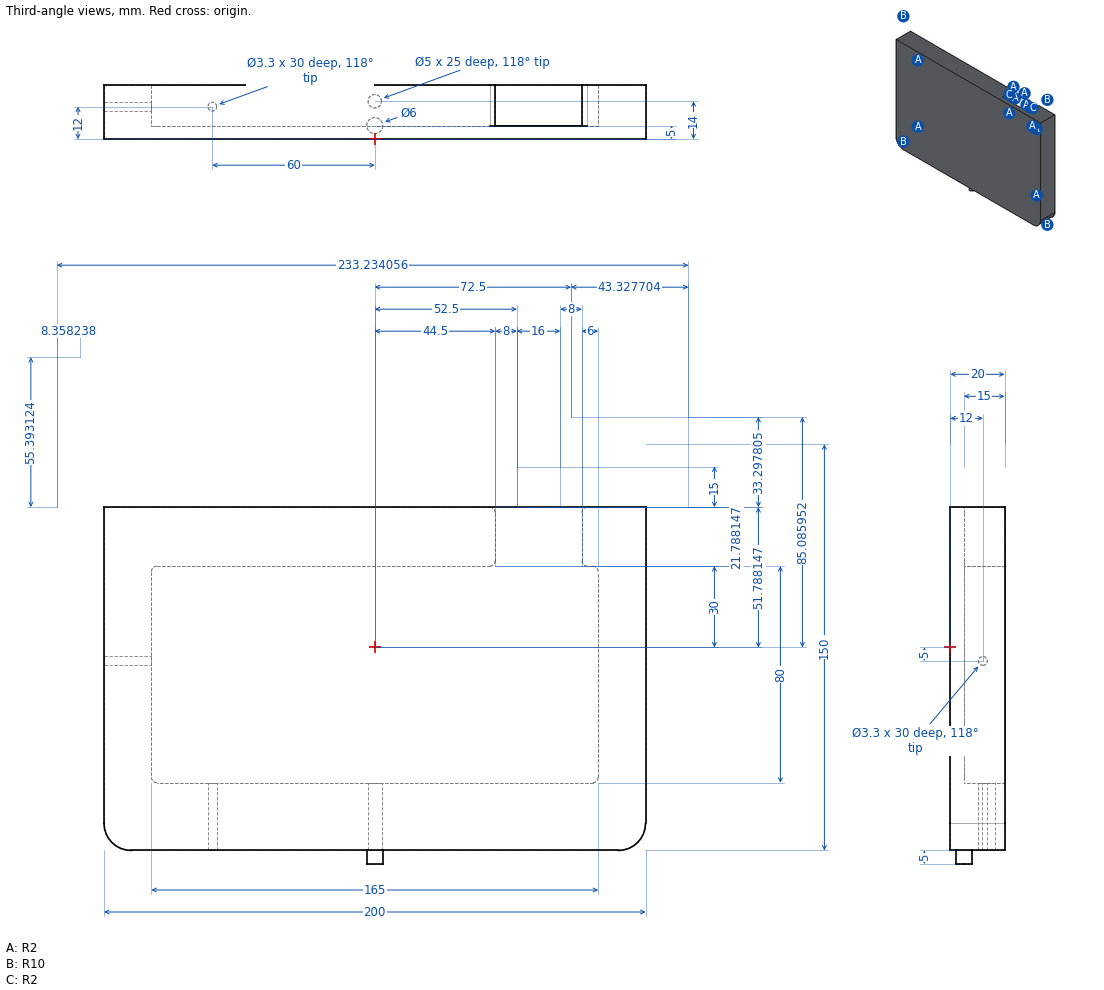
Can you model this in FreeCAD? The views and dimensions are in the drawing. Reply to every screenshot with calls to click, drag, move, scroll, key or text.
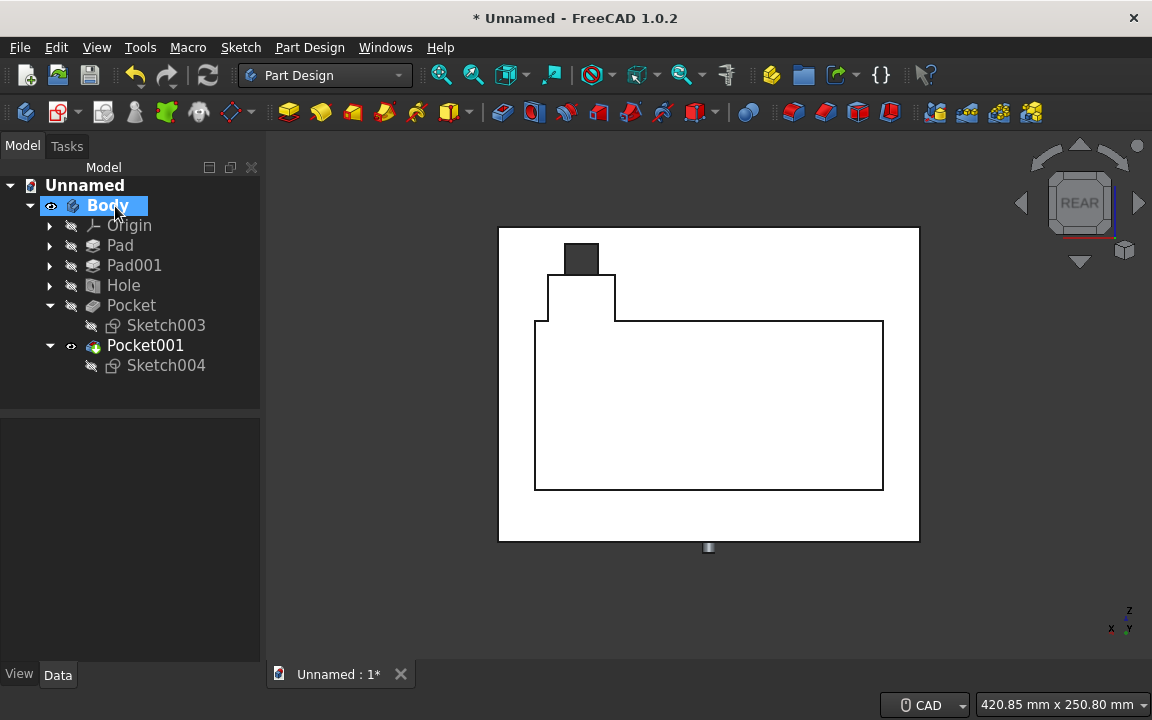
key(6)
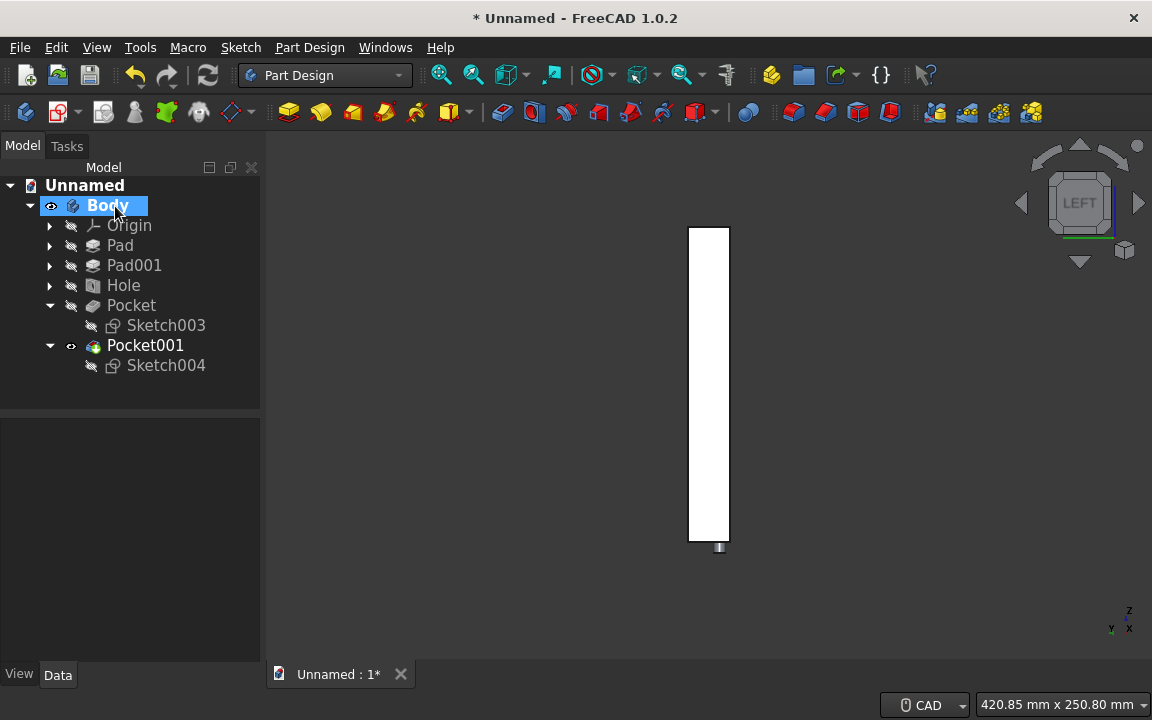
key(v)
key(3)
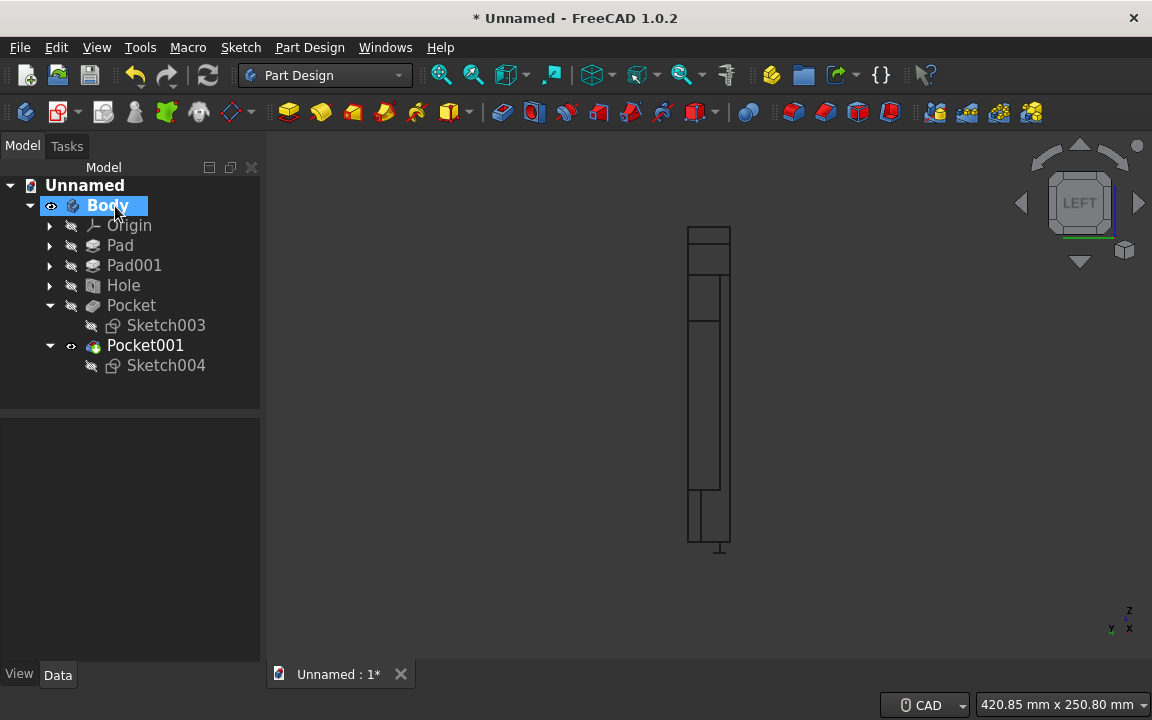
key(0)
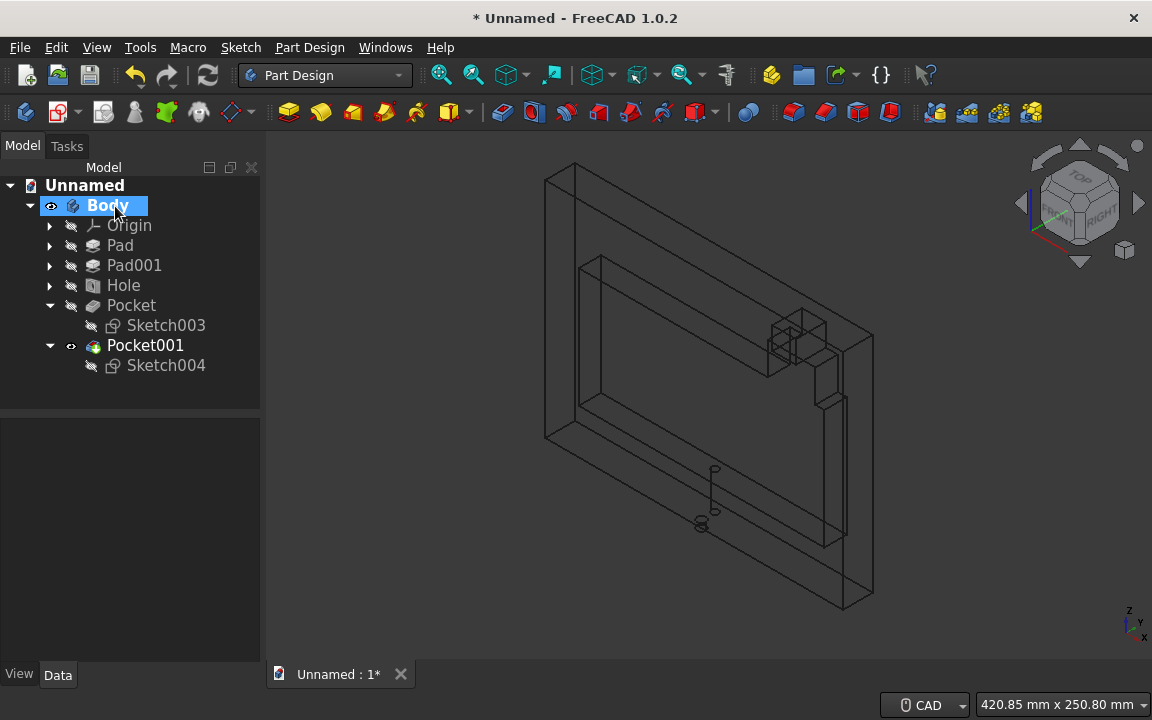
click(590, 398)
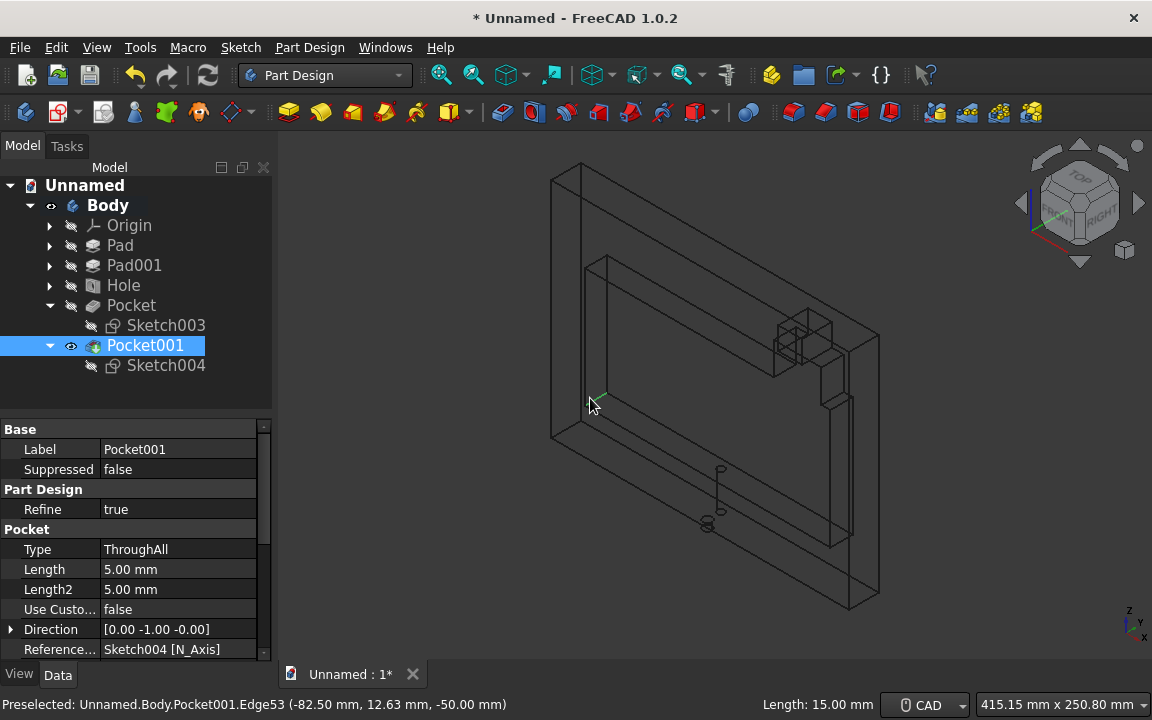
click(596, 261, ctrl)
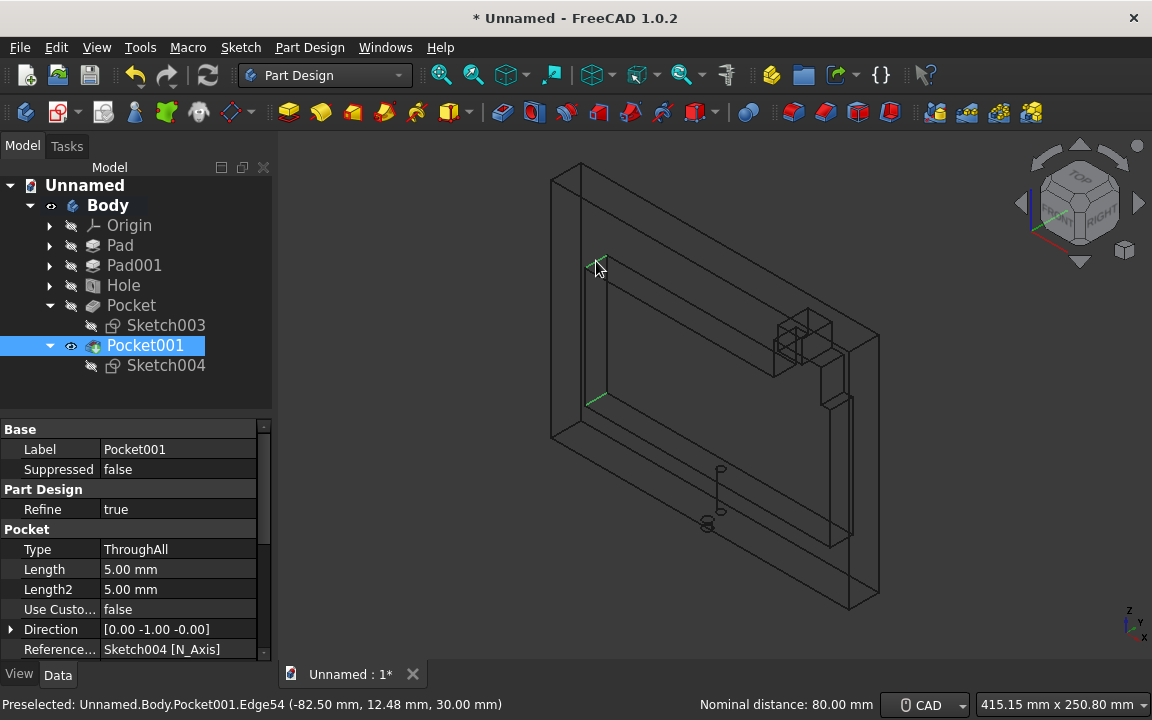
click(842, 540, ctrl)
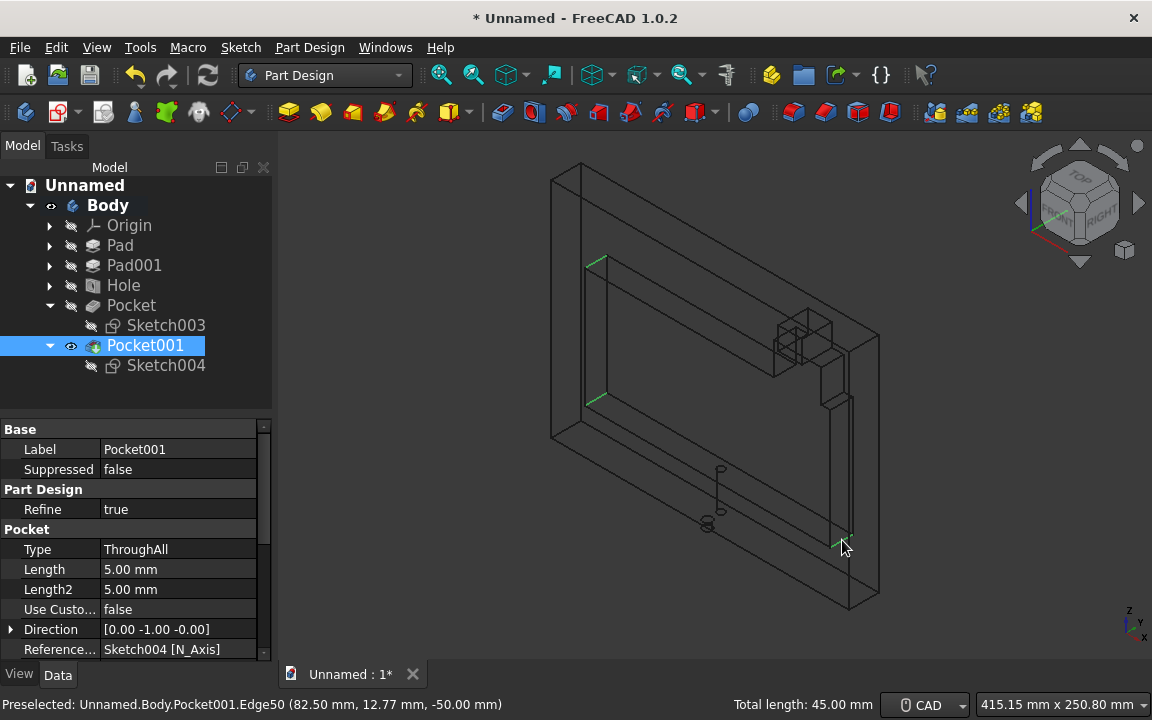
click(842, 403, ctrl)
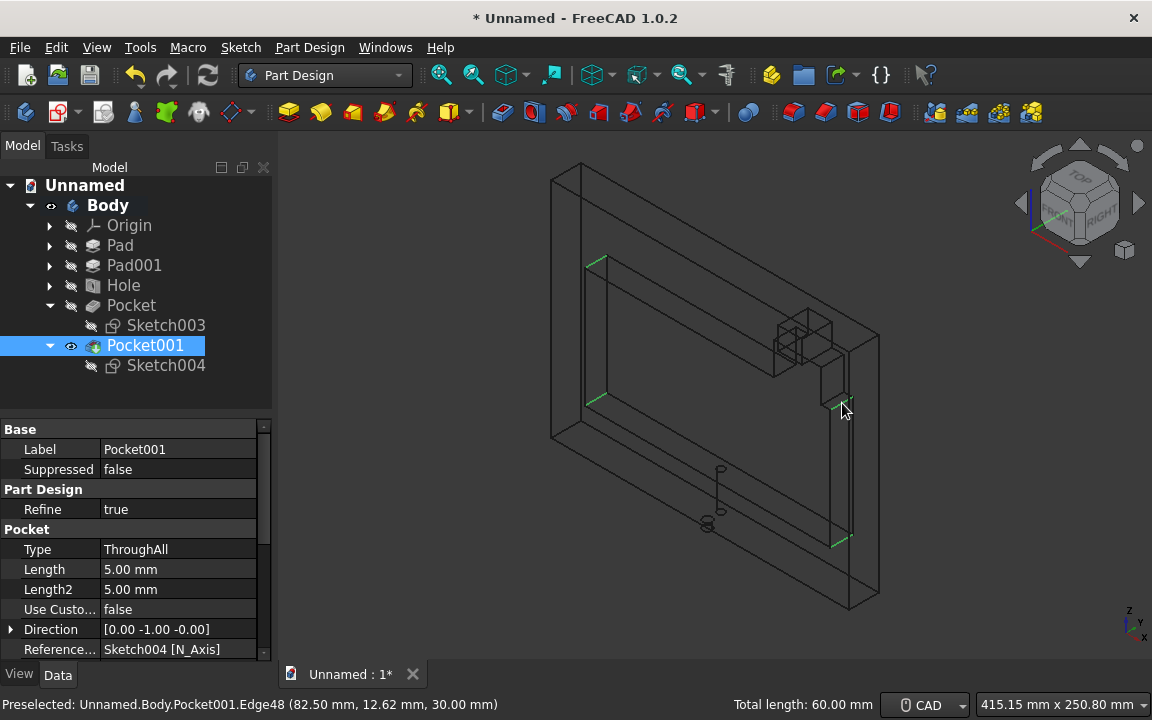
click(833, 397, ctrl)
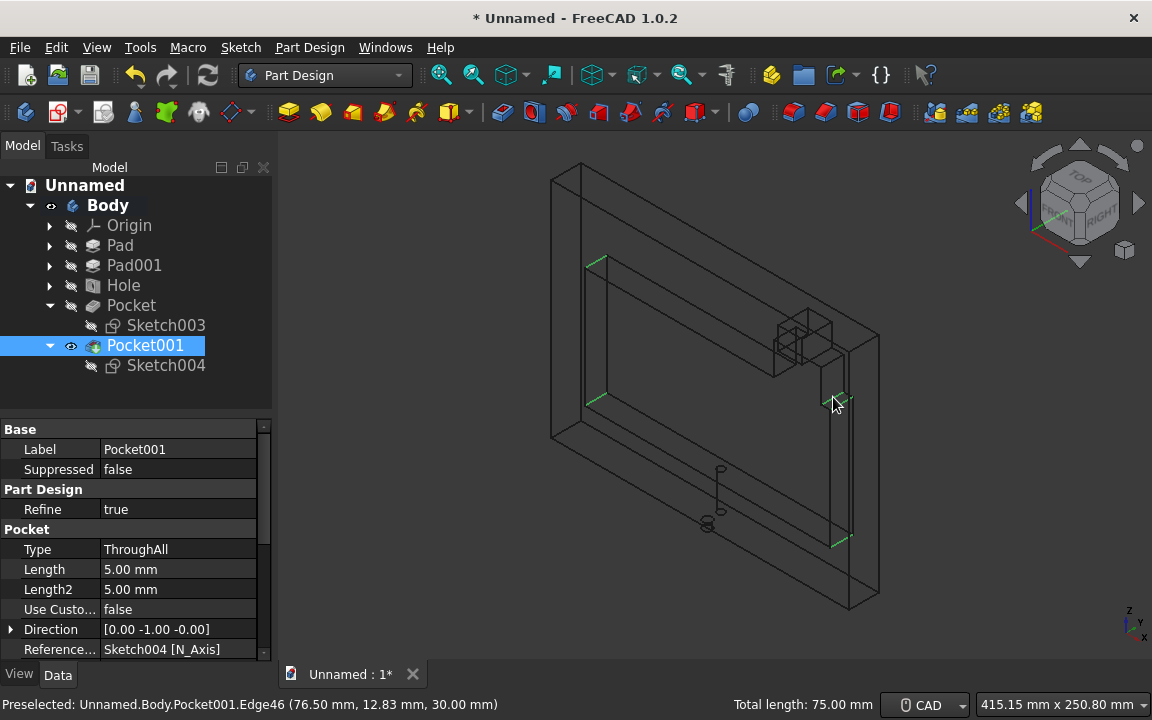
click(821, 353, ctrl)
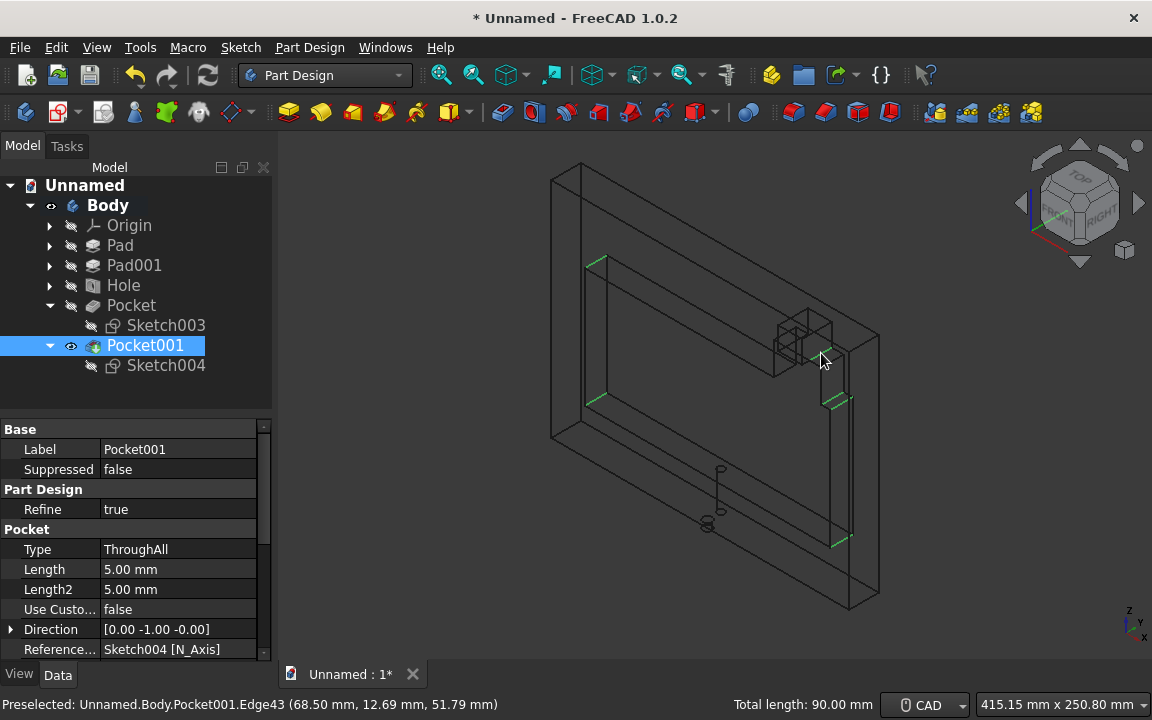
click(823, 326, ctrl)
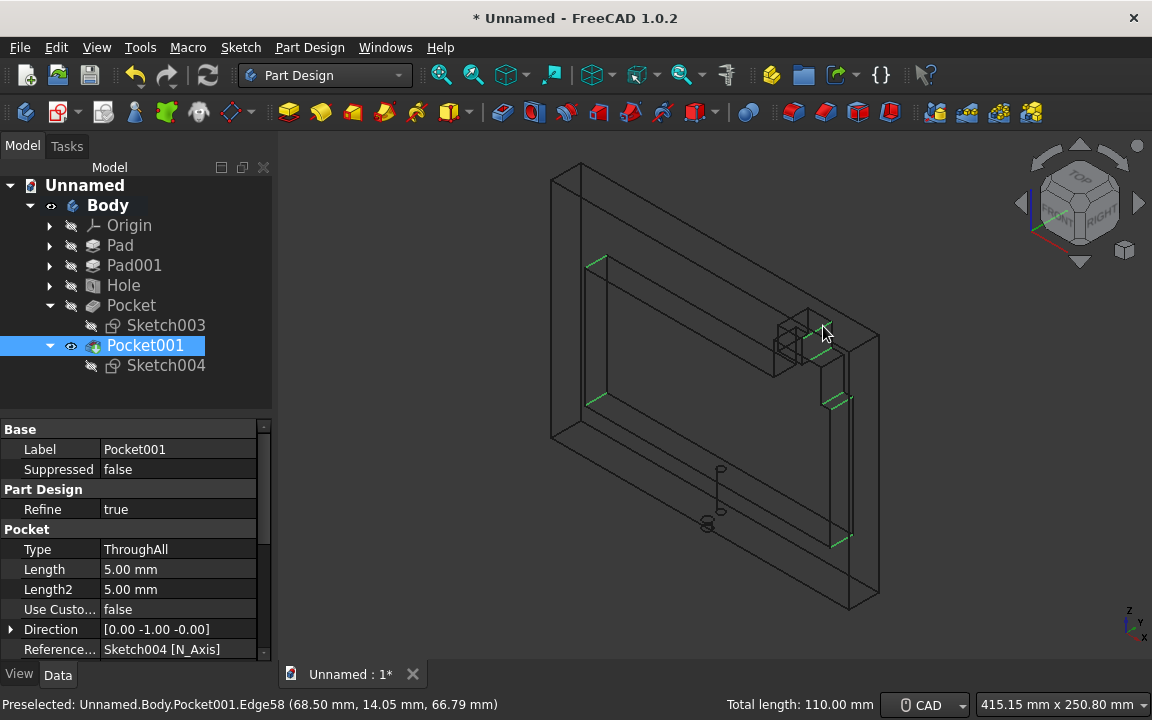
click(799, 312, ctrl)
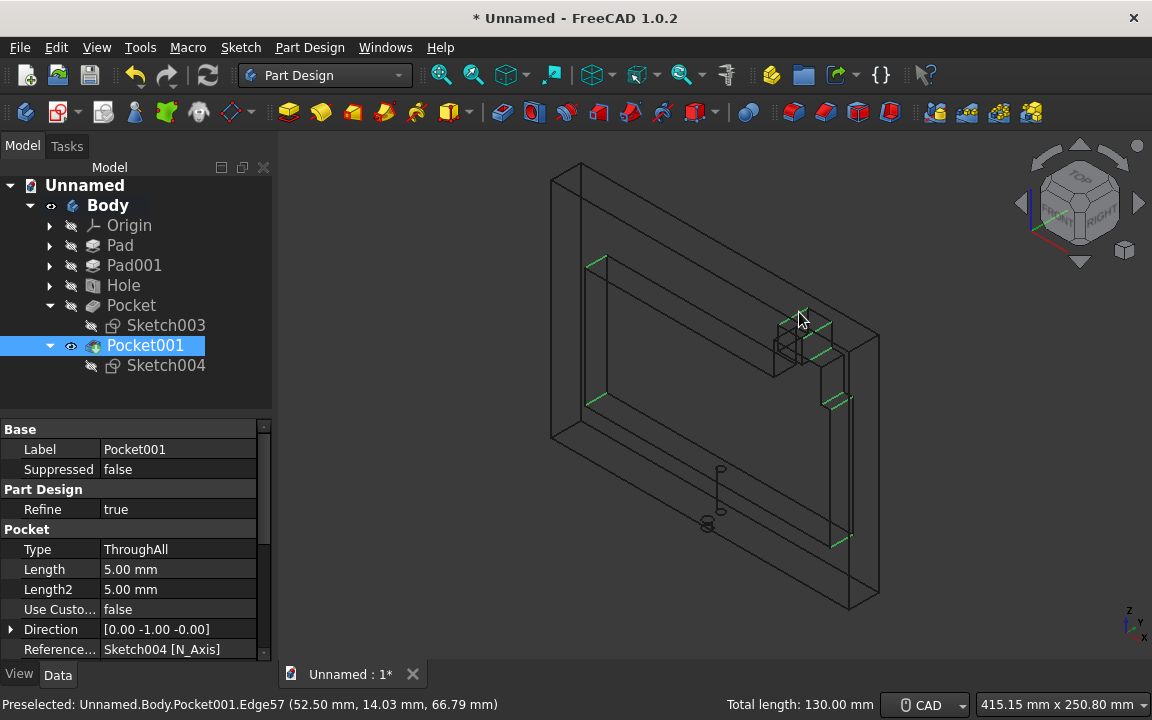
click(792, 342, ctrl)